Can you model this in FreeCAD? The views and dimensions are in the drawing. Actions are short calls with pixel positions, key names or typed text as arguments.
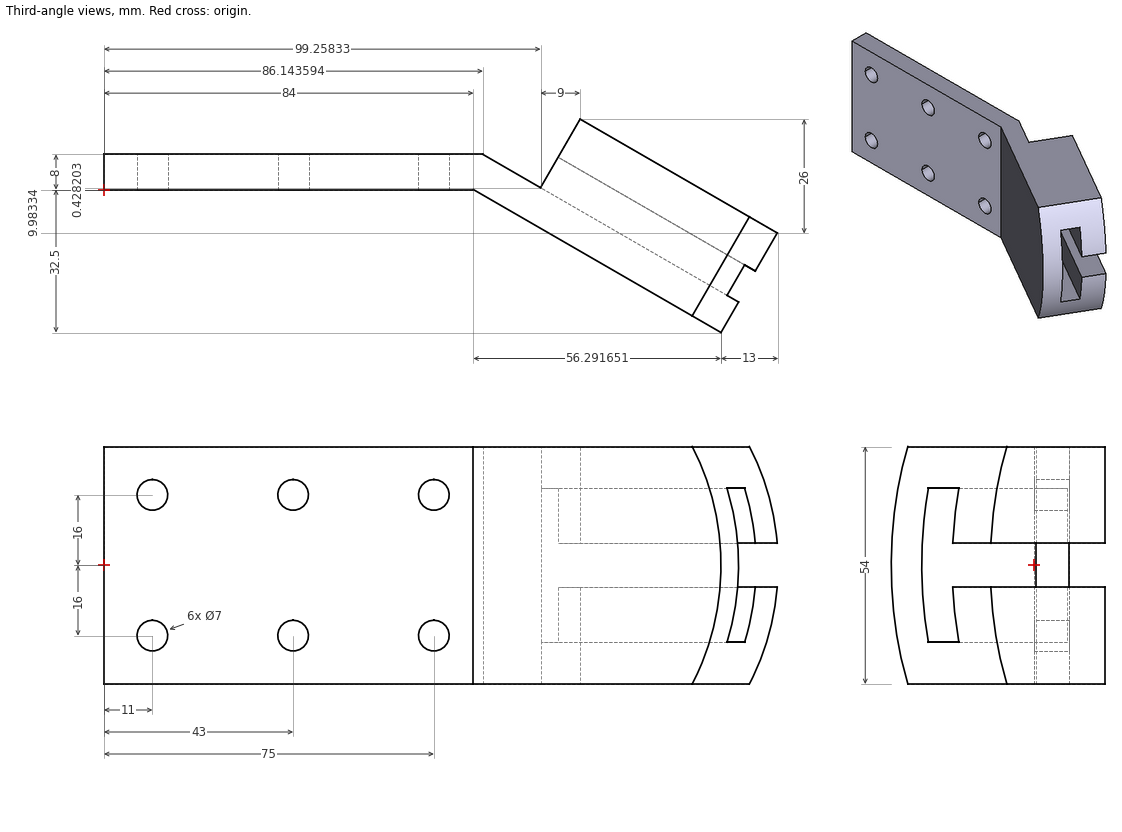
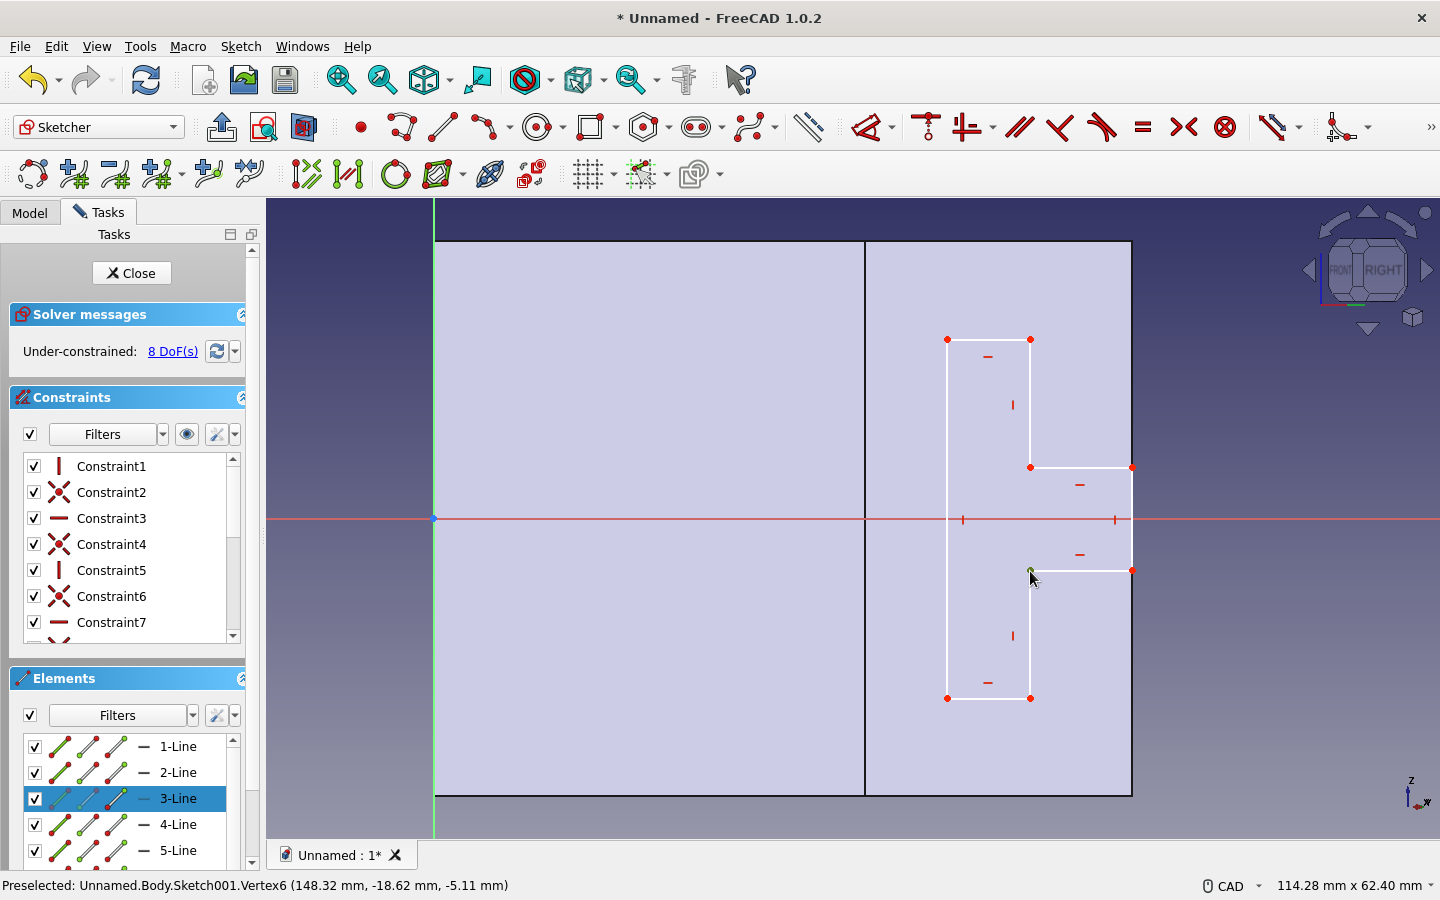
click(1030, 468)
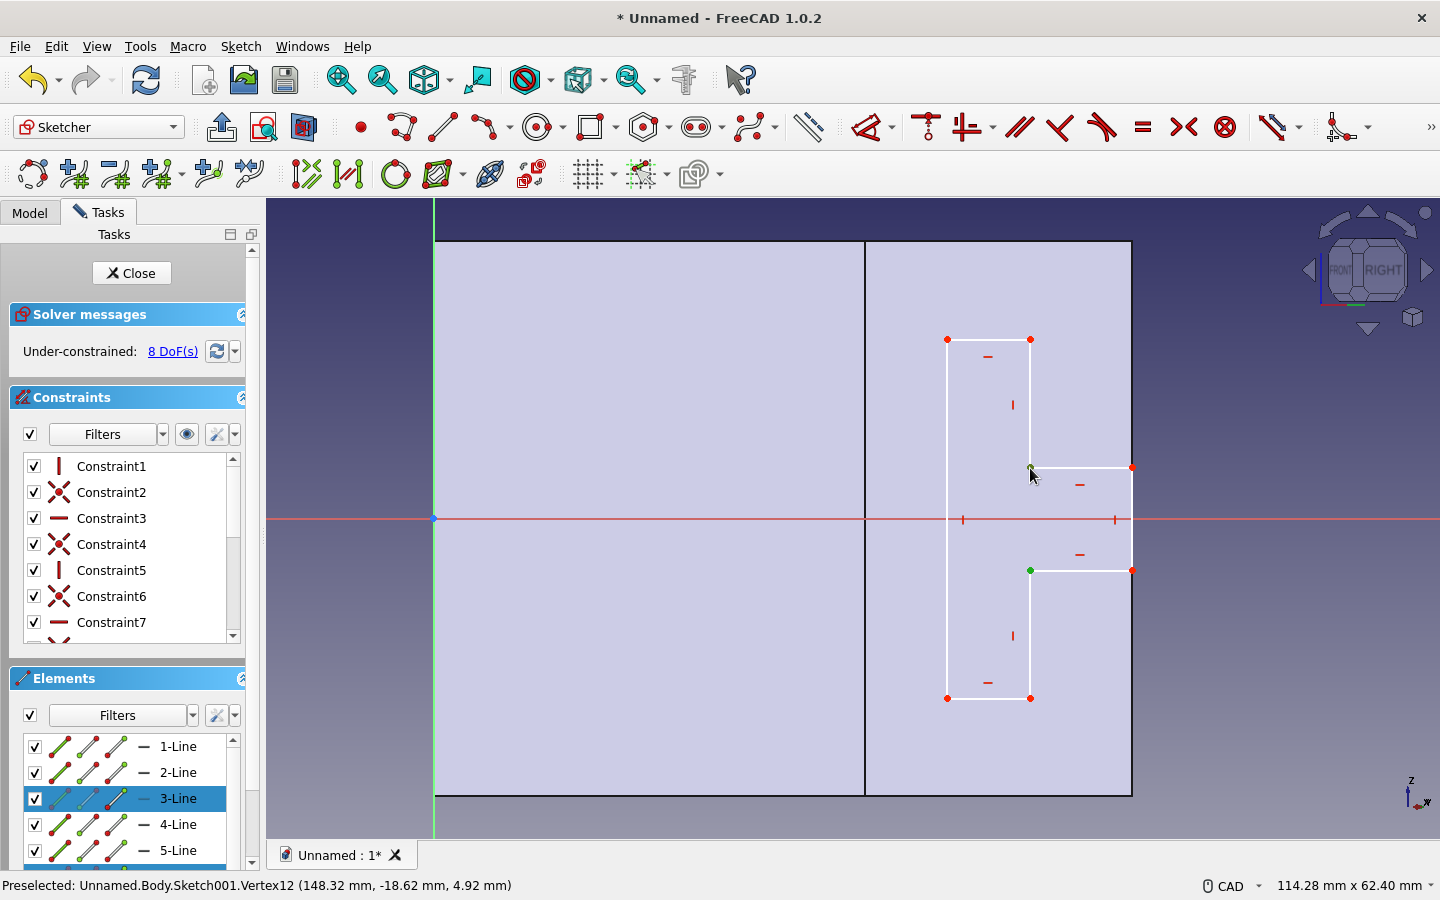
click(364, 518)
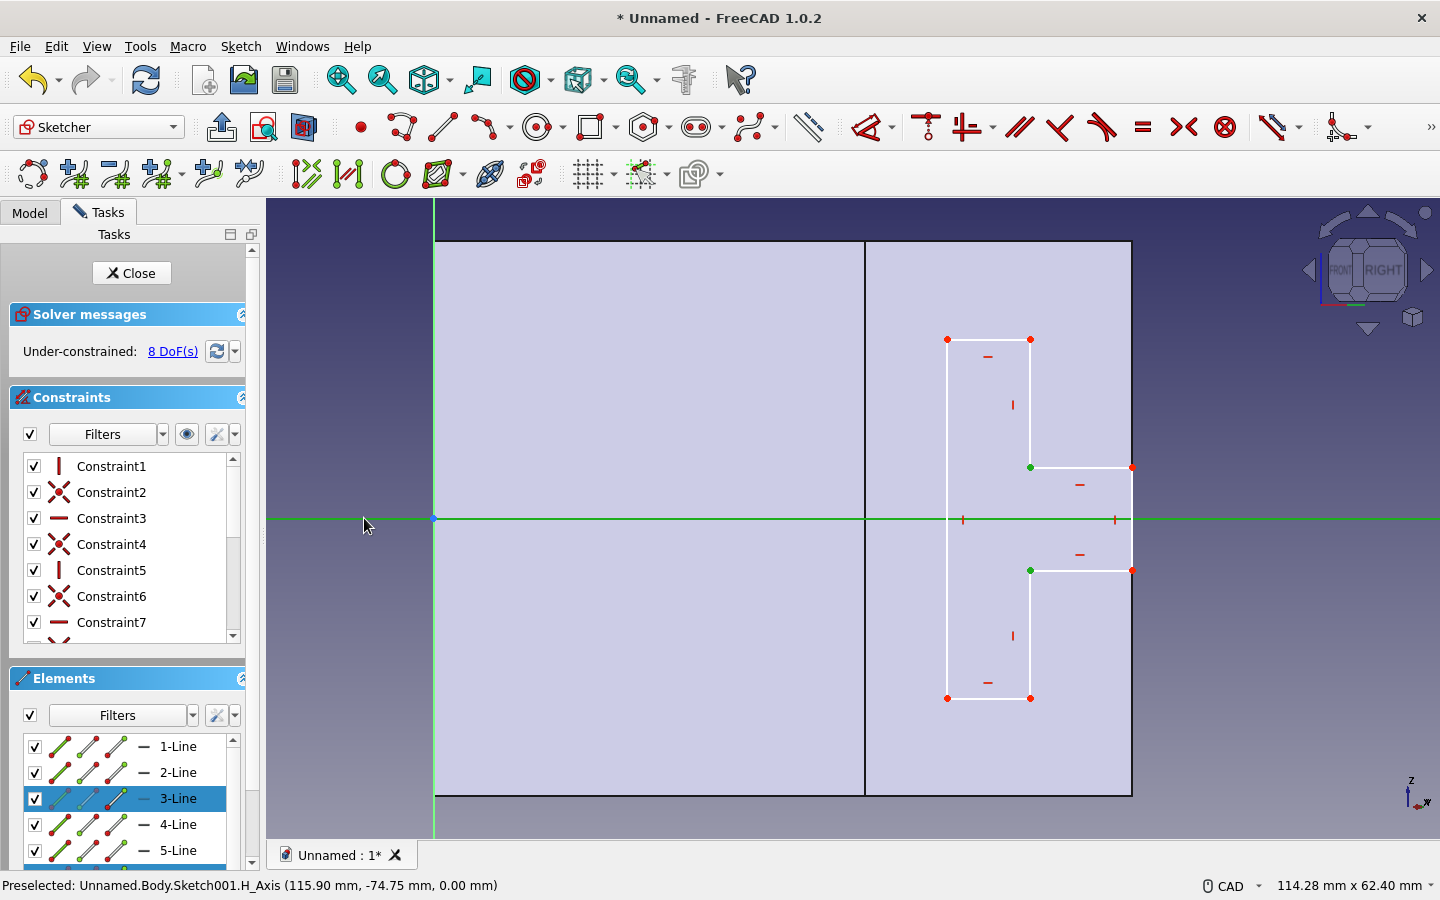
key(s)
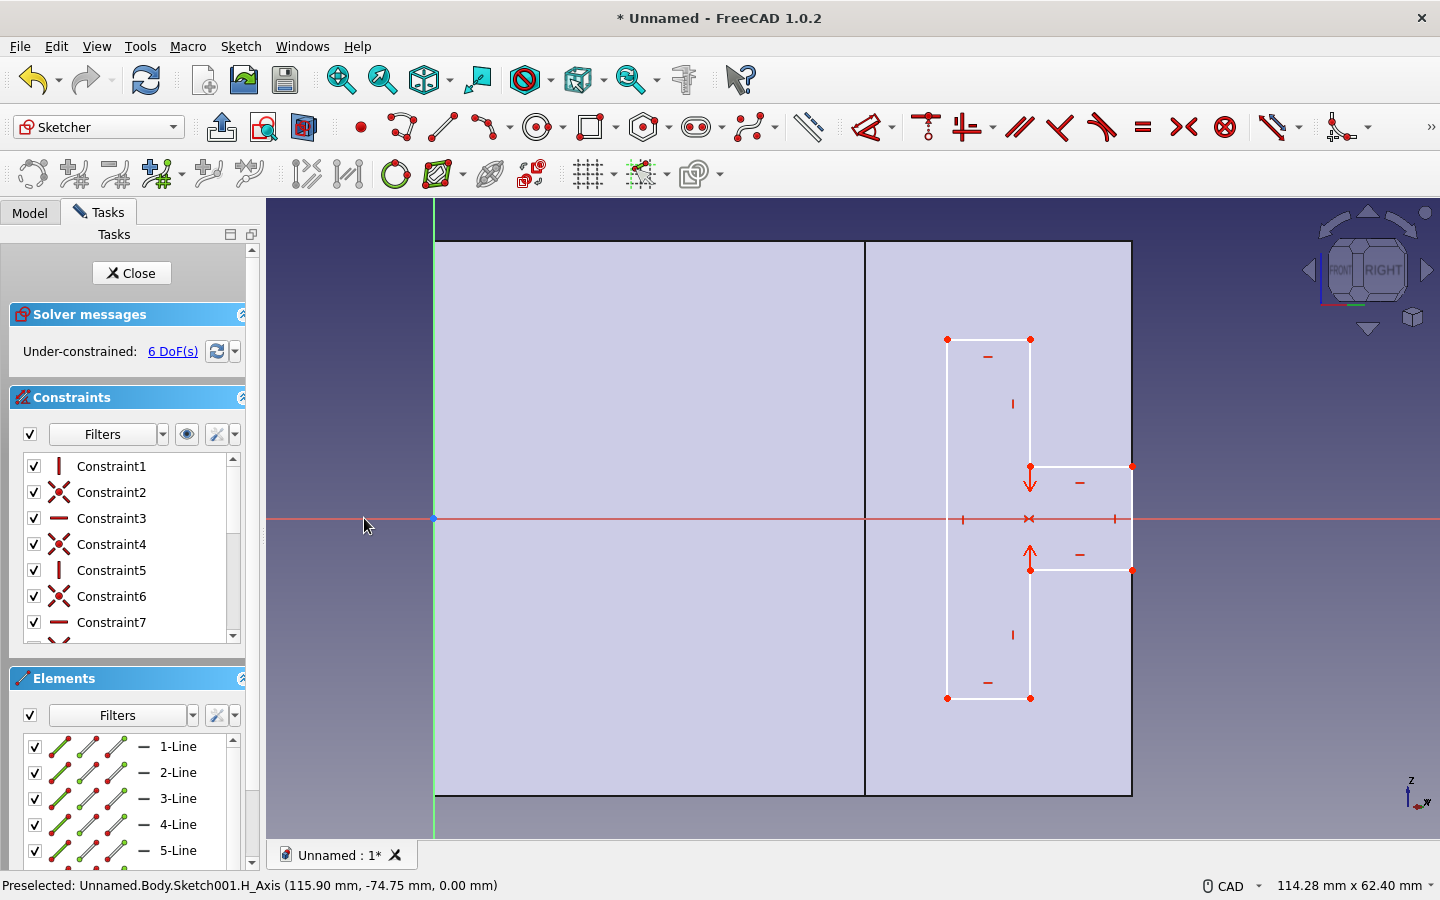
key(d)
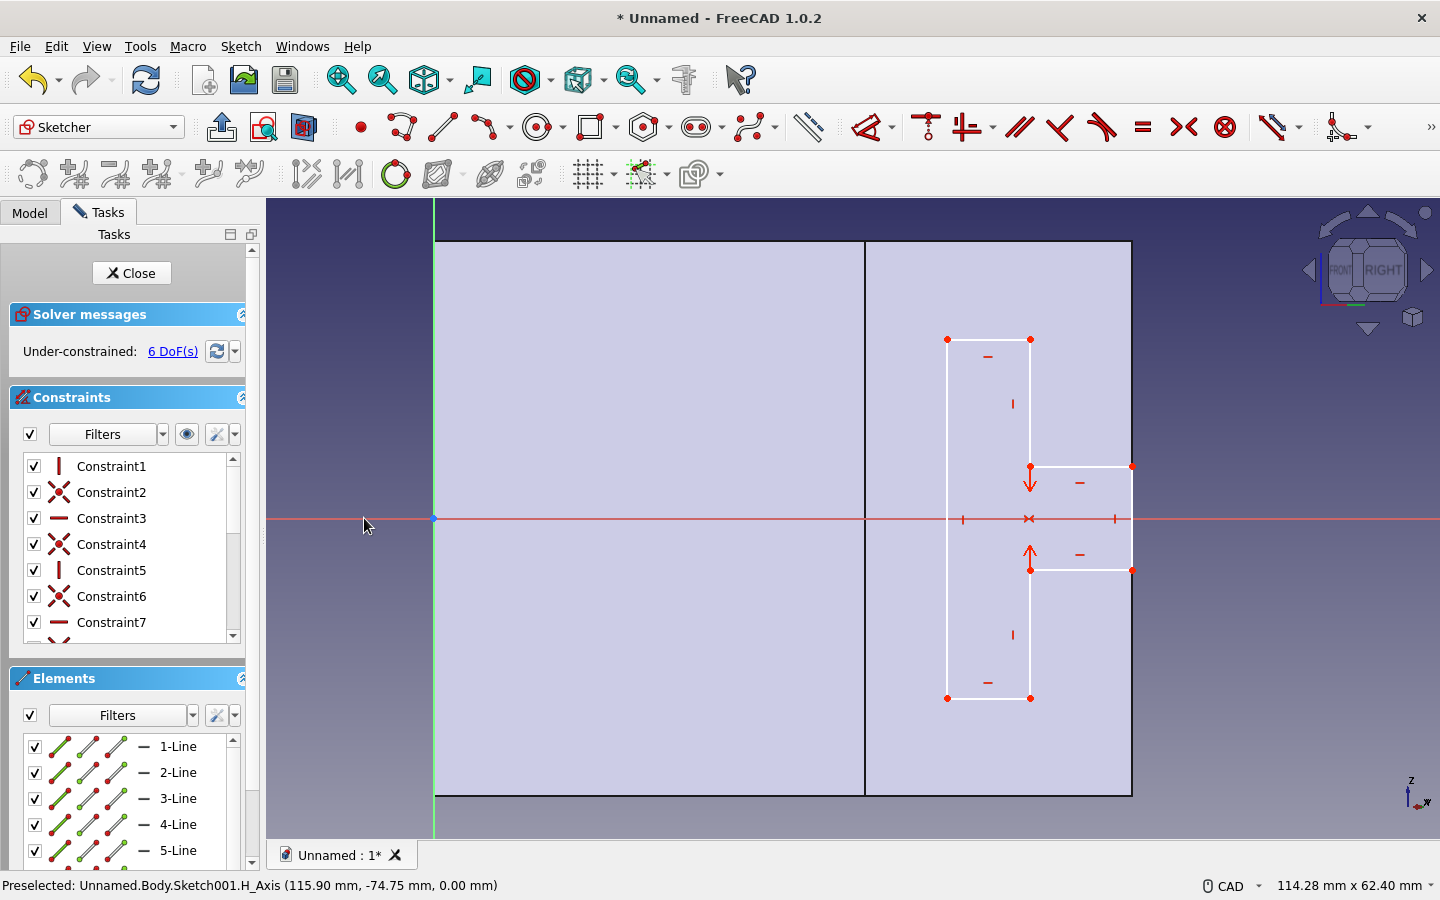
click(972, 699)
click(989, 733)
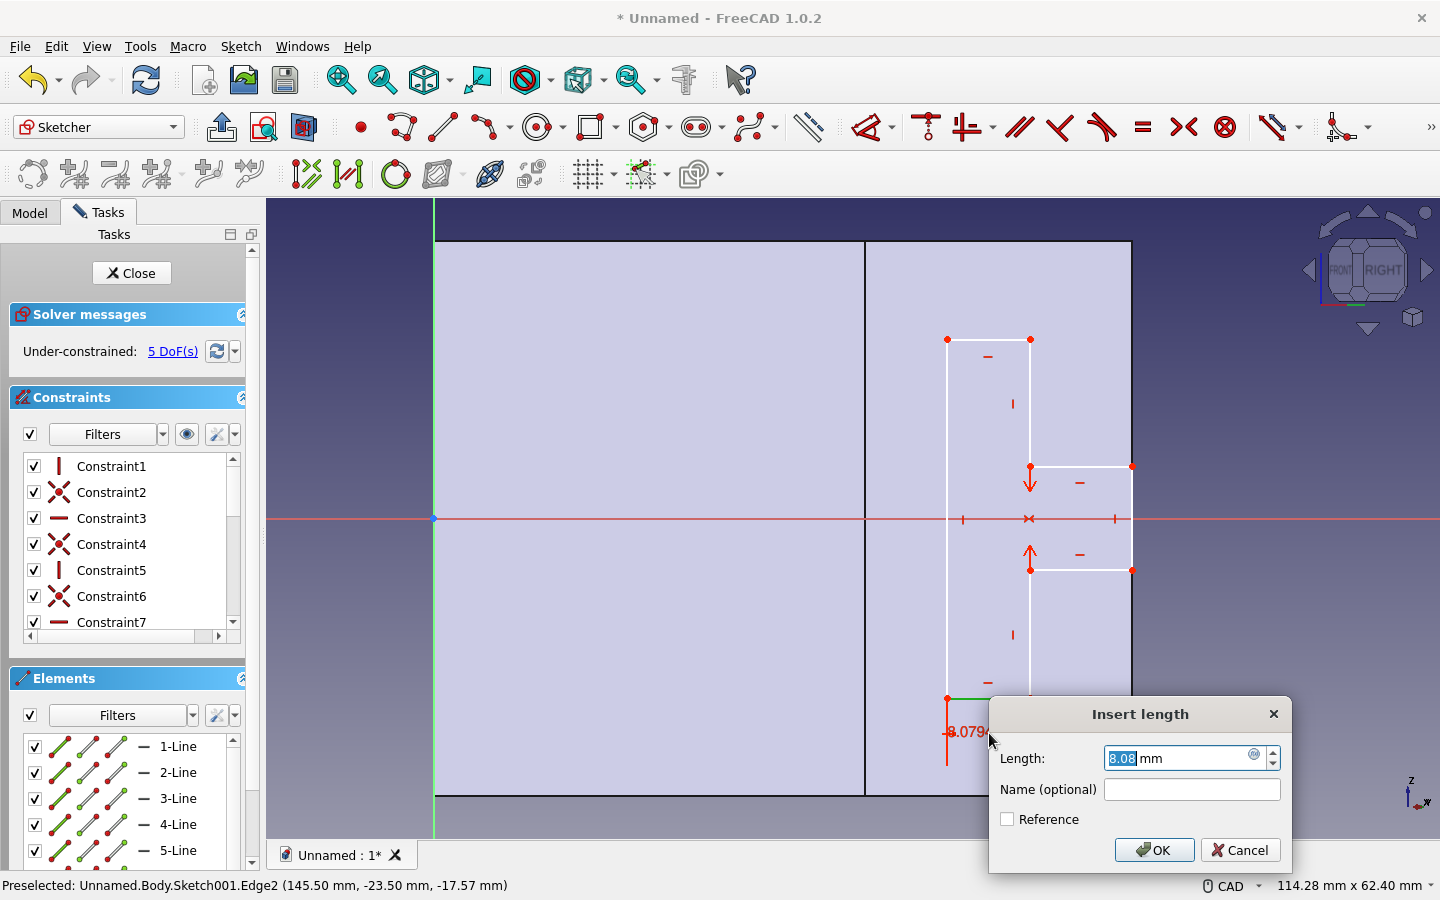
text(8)
key(Return)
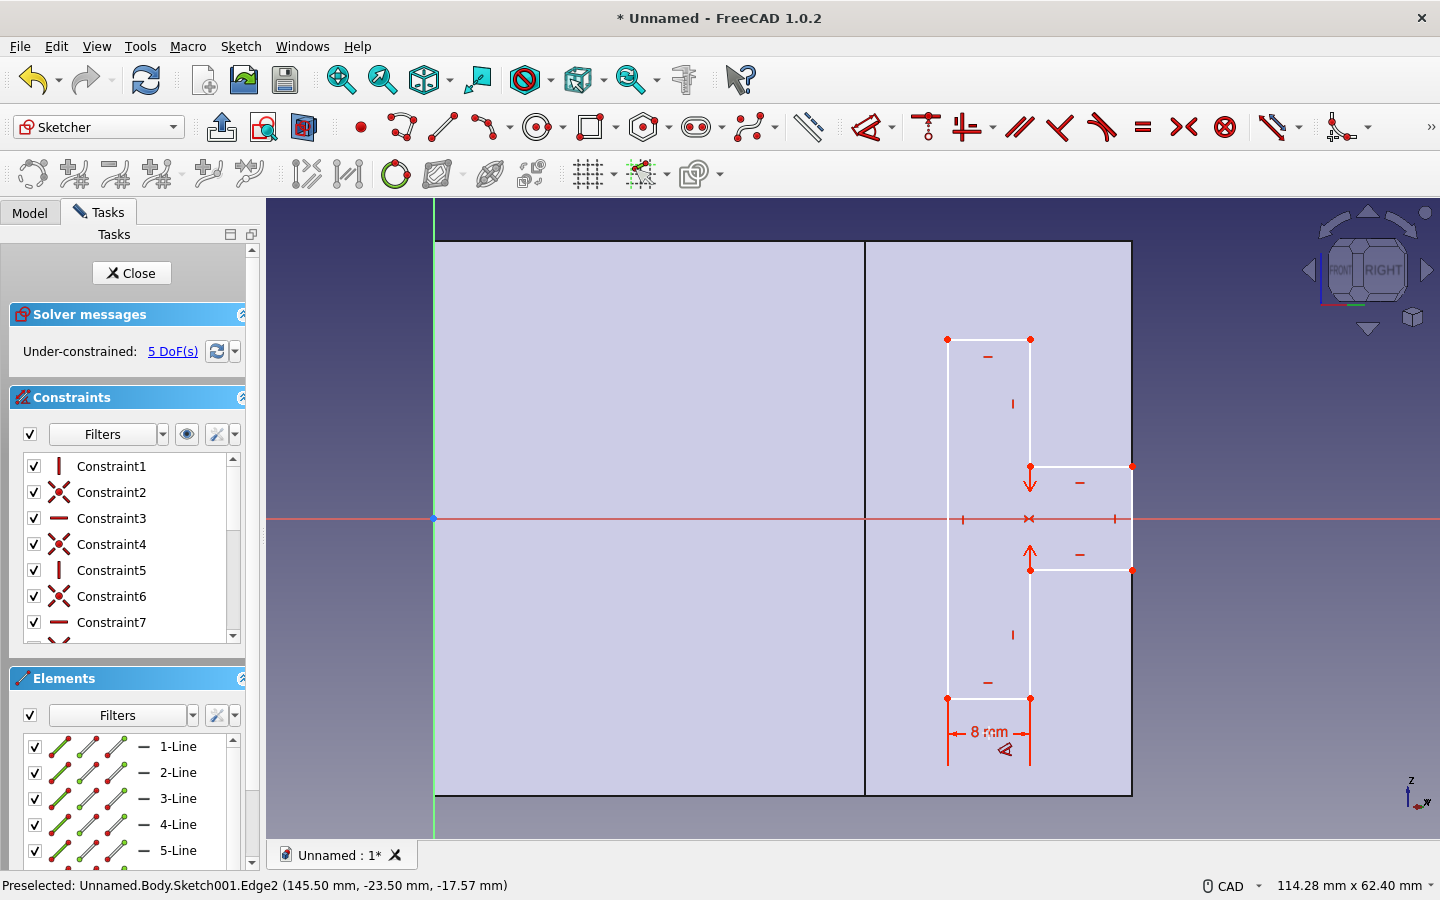
click(948, 448)
click(982, 437)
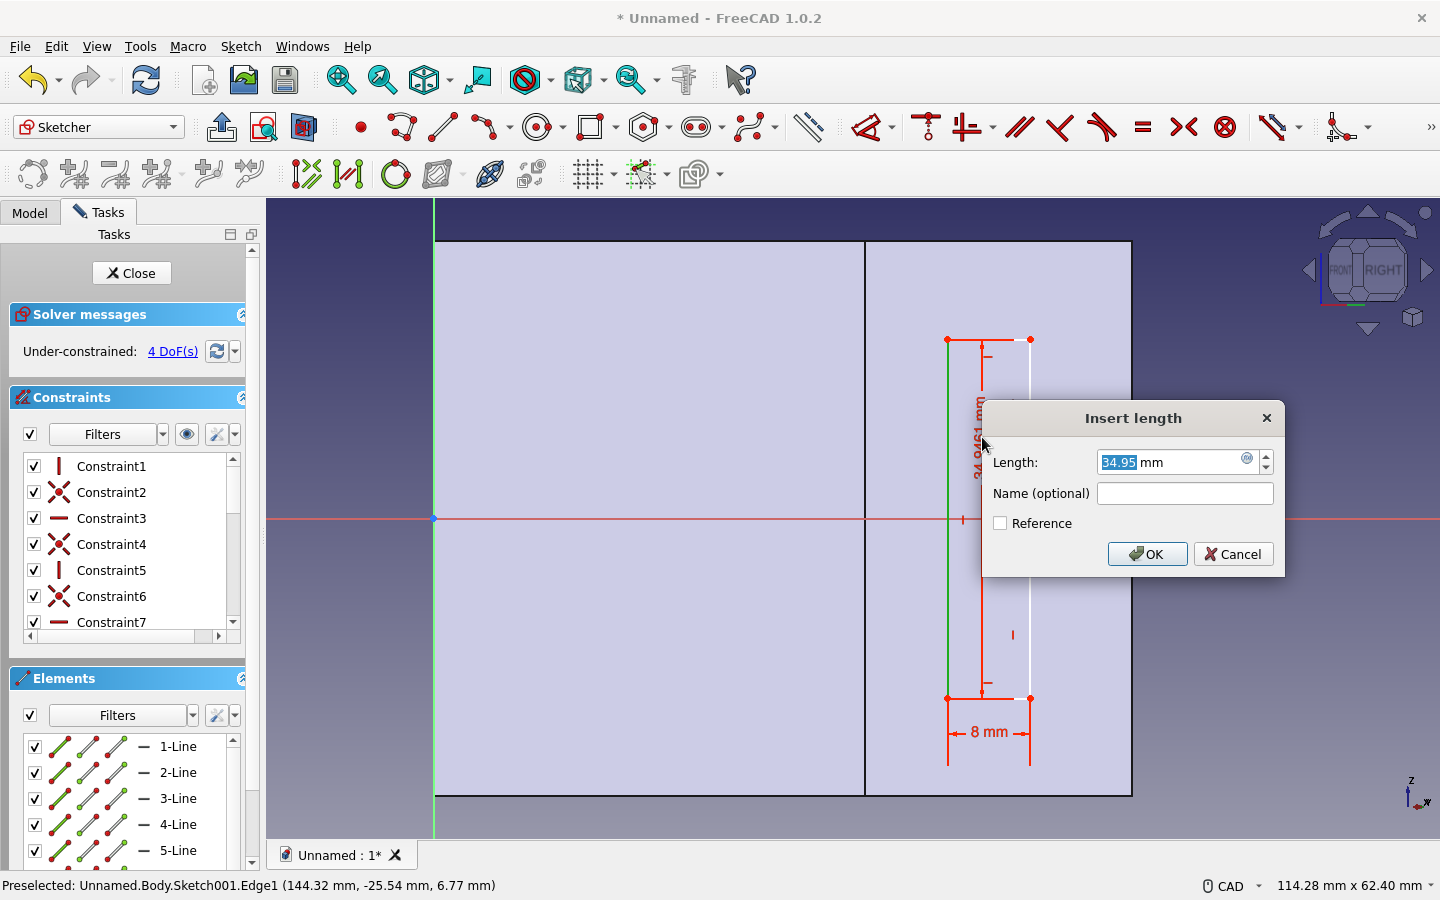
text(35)
key(Return)